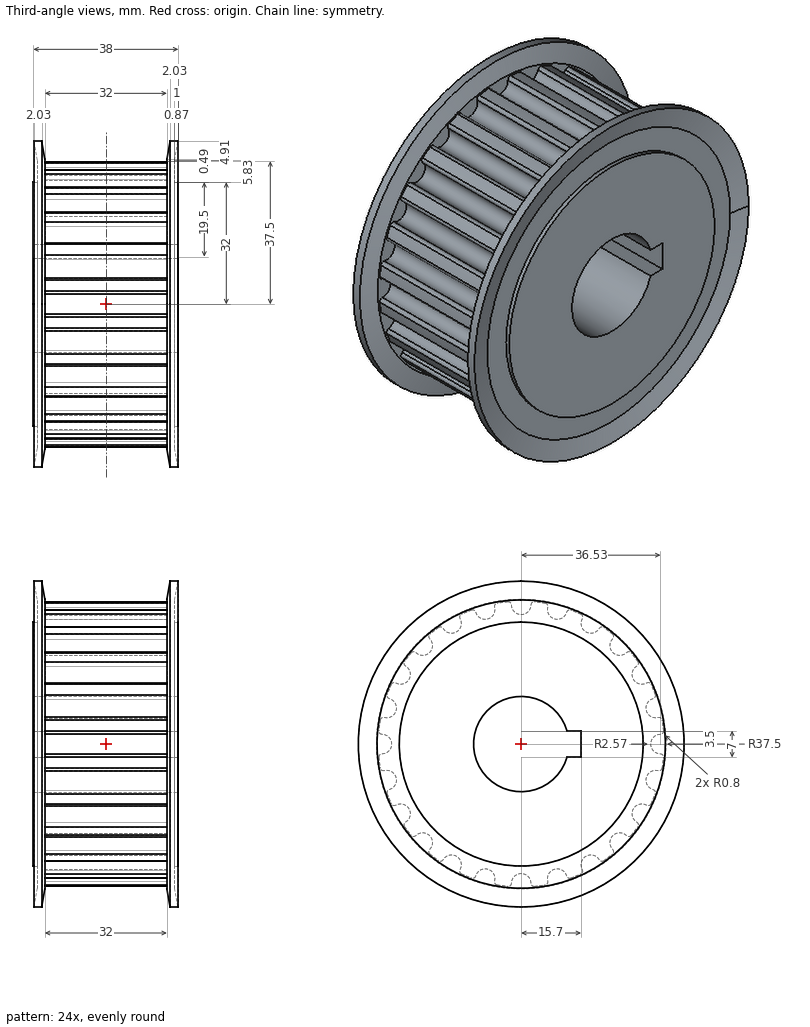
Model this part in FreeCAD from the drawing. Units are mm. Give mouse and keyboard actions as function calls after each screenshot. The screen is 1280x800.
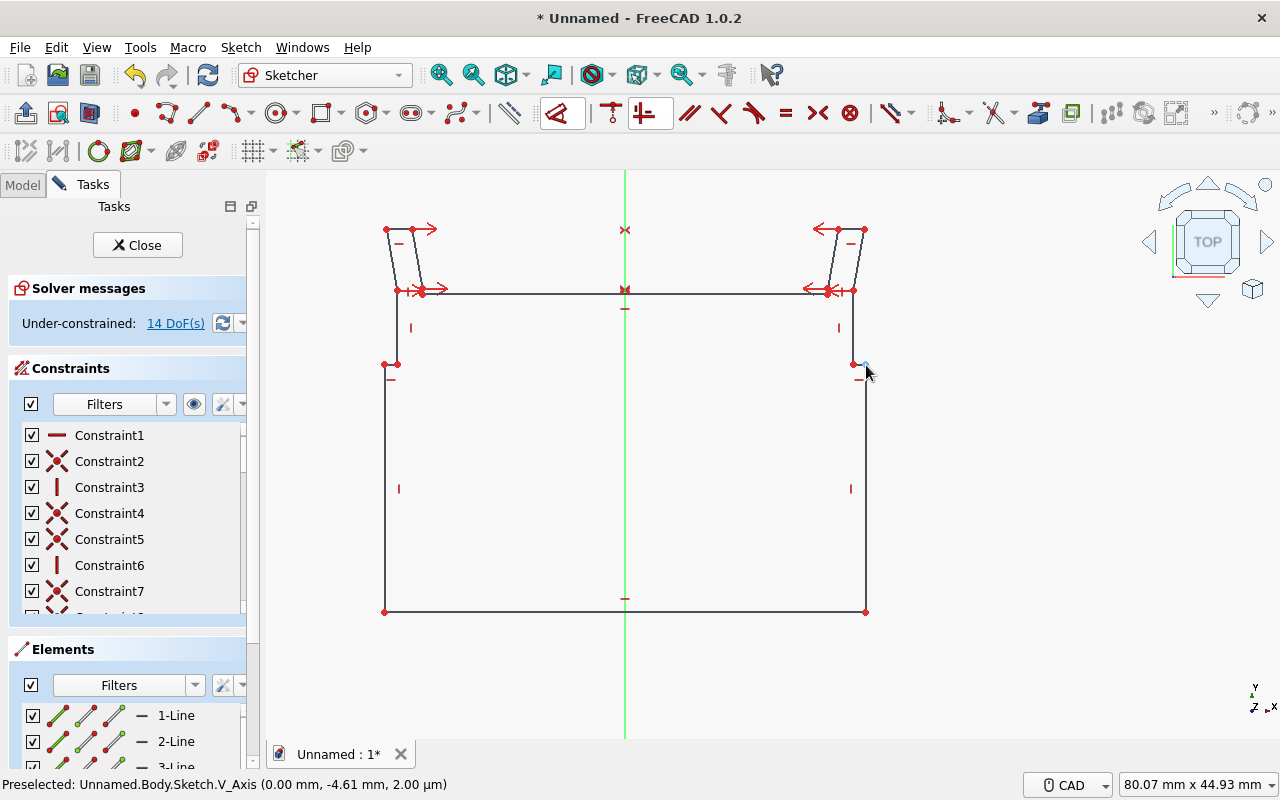
click(866, 365)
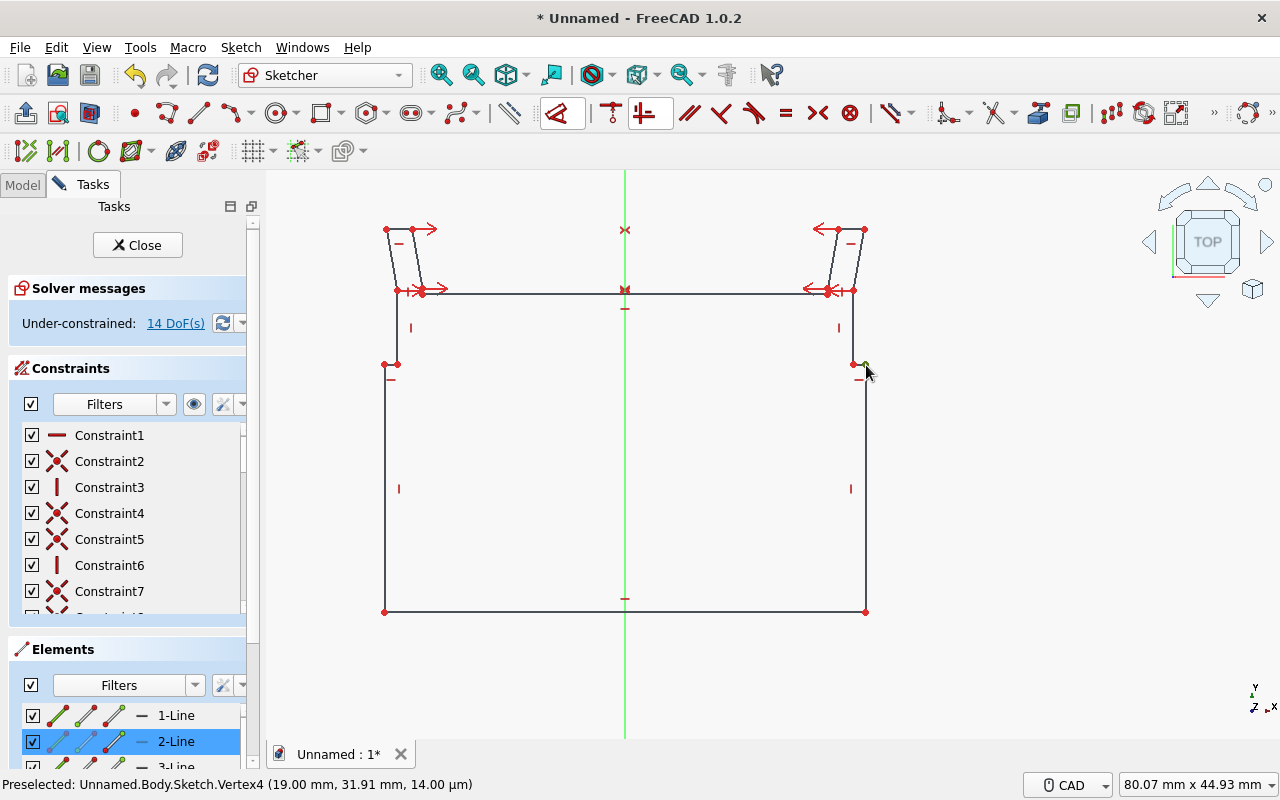
click(385, 365)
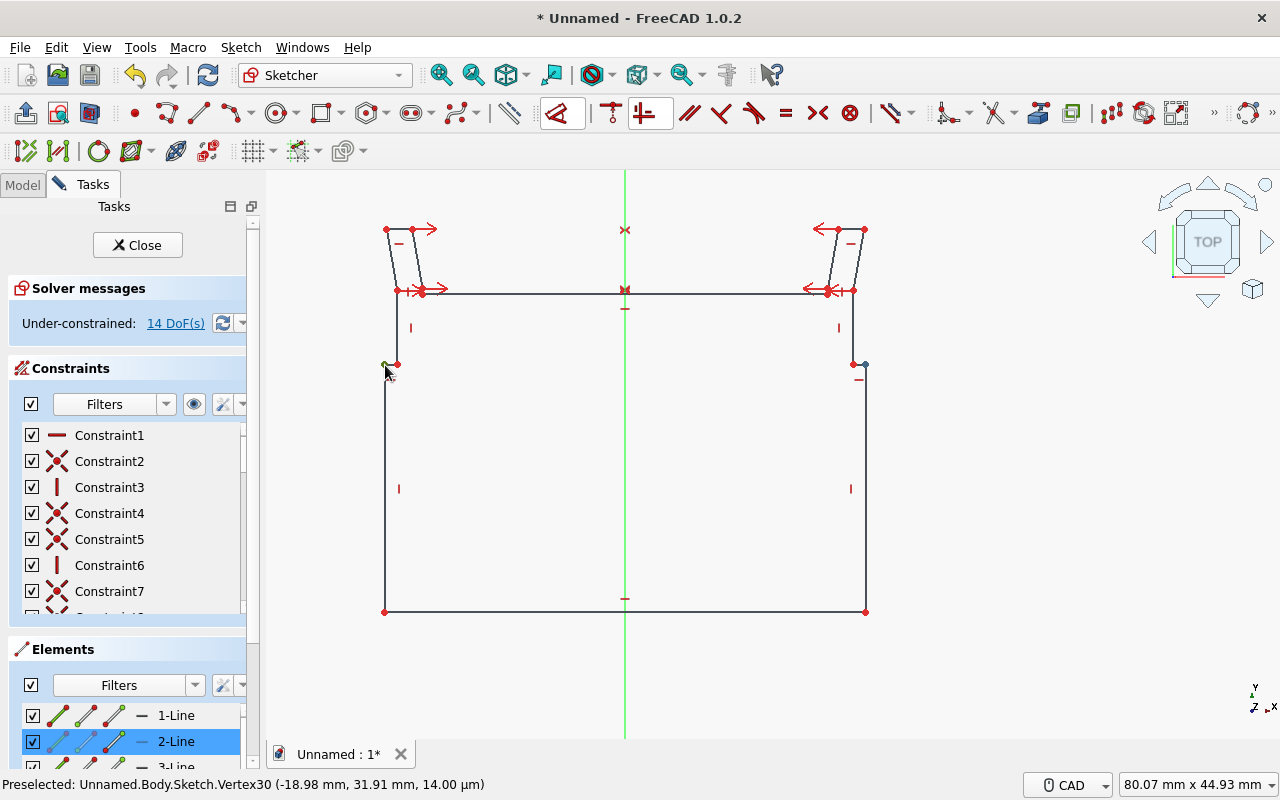
click(625, 674)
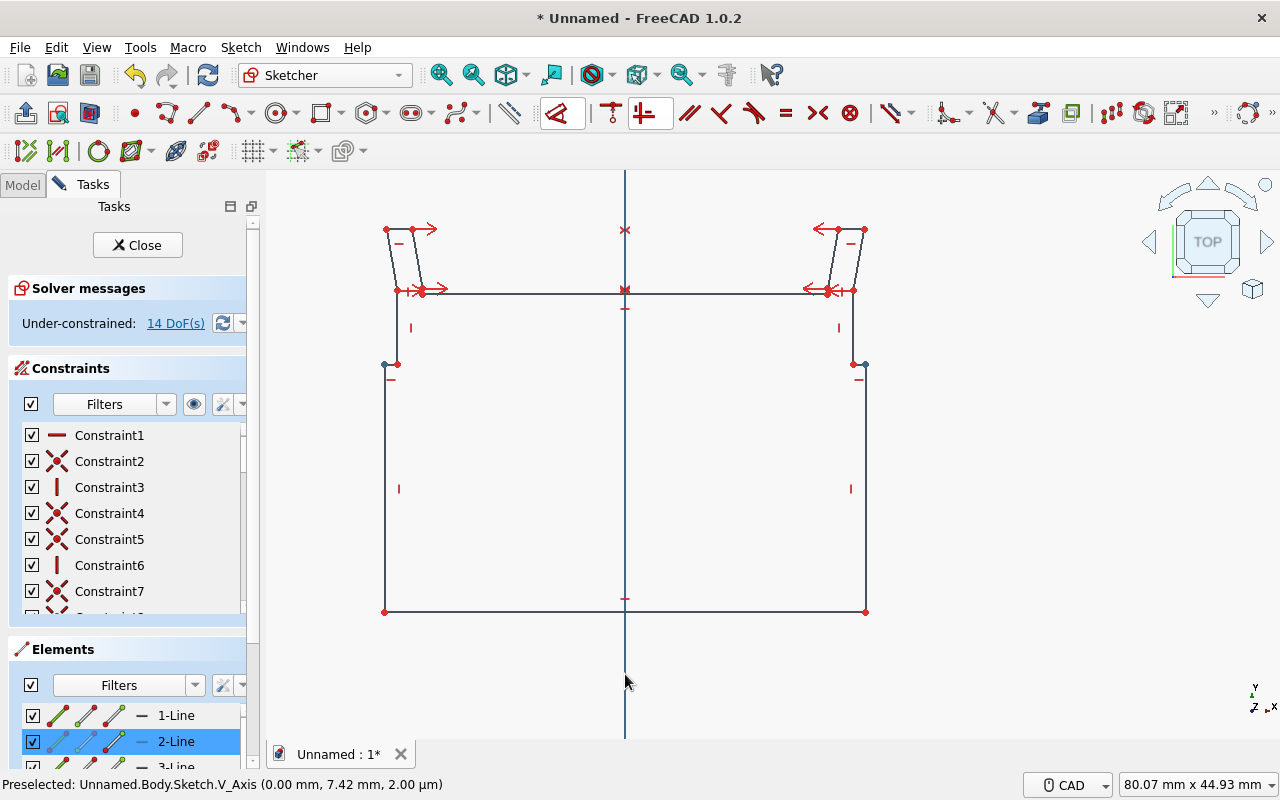
click(818, 114)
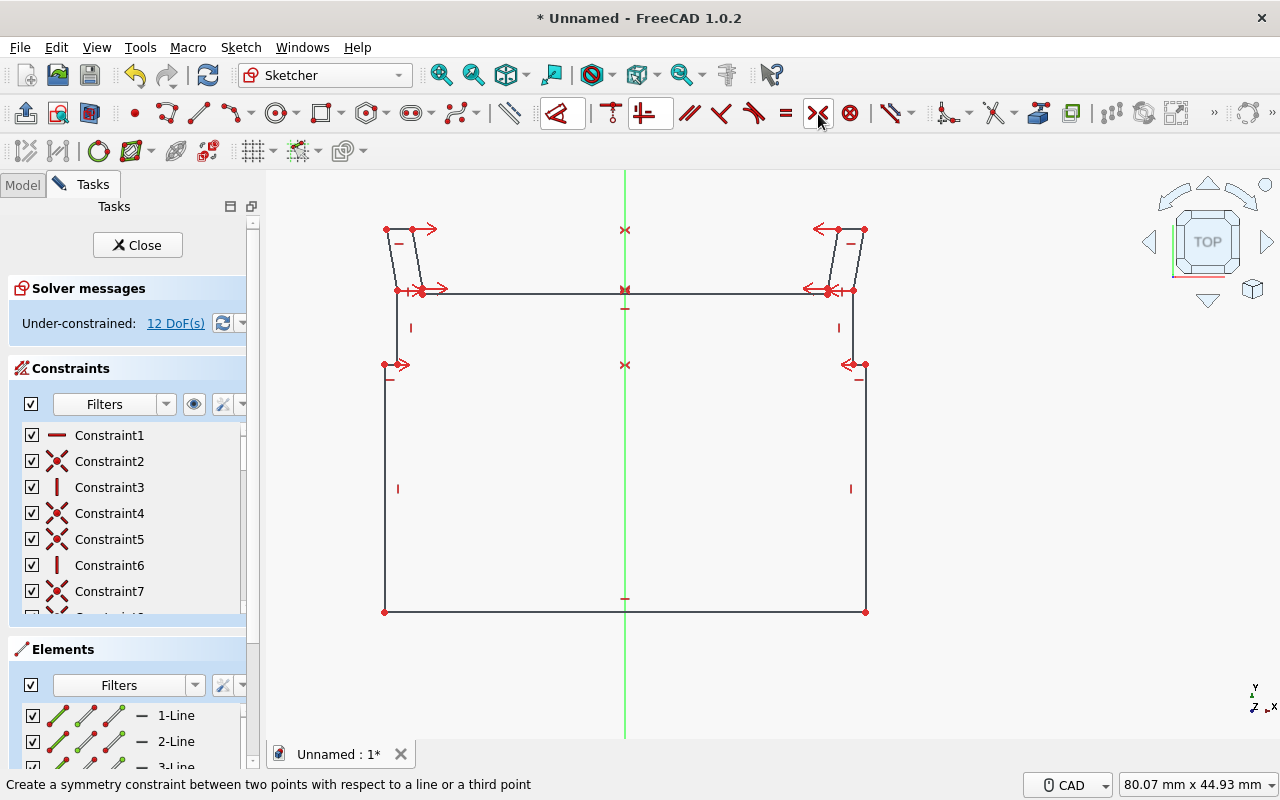
click(556, 114)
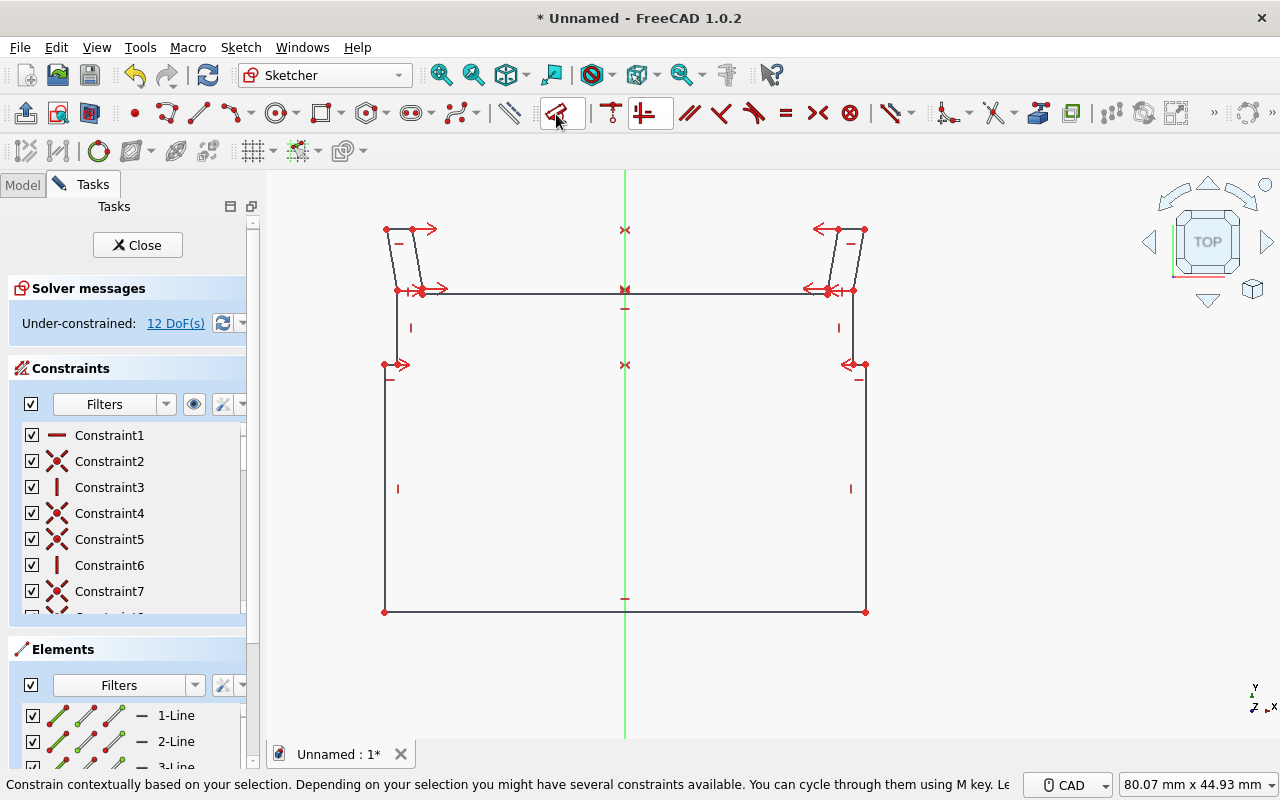
scroll(860, 365, up, 6)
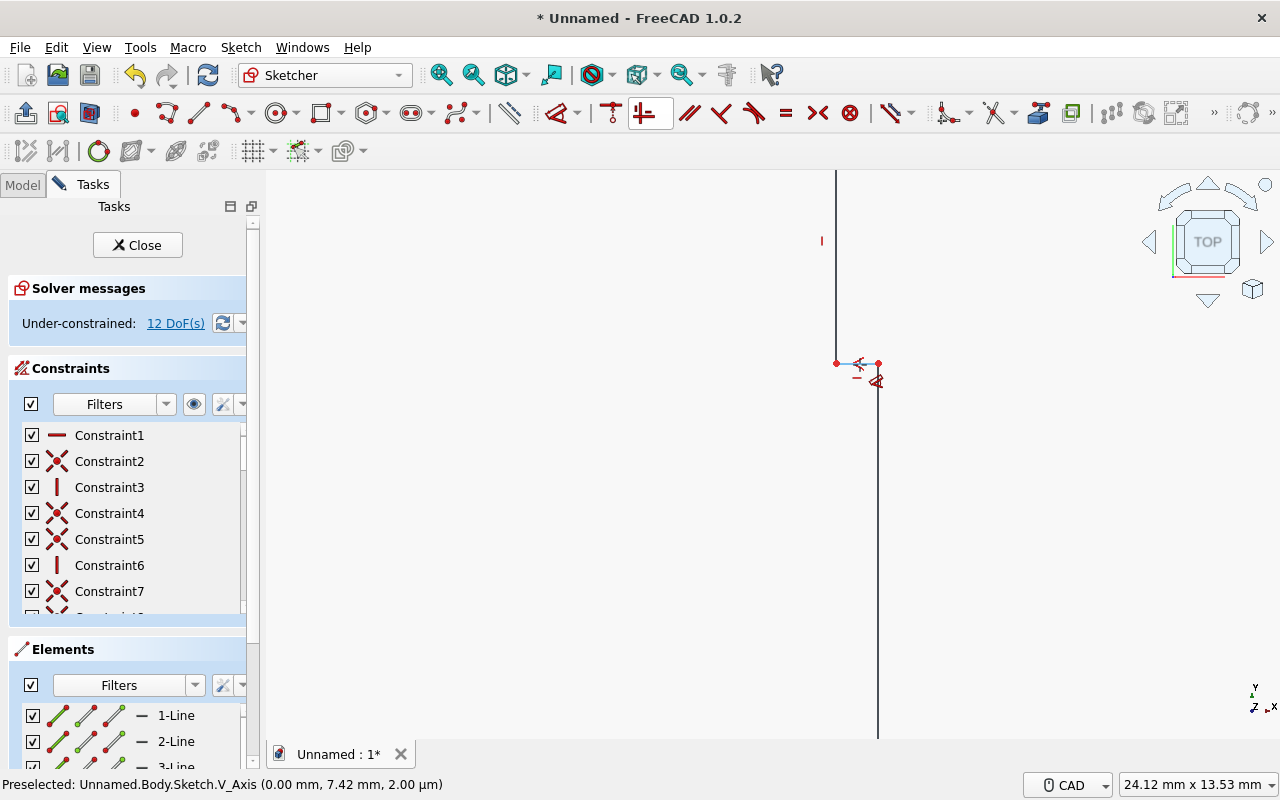
click(857, 364)
click(857, 330)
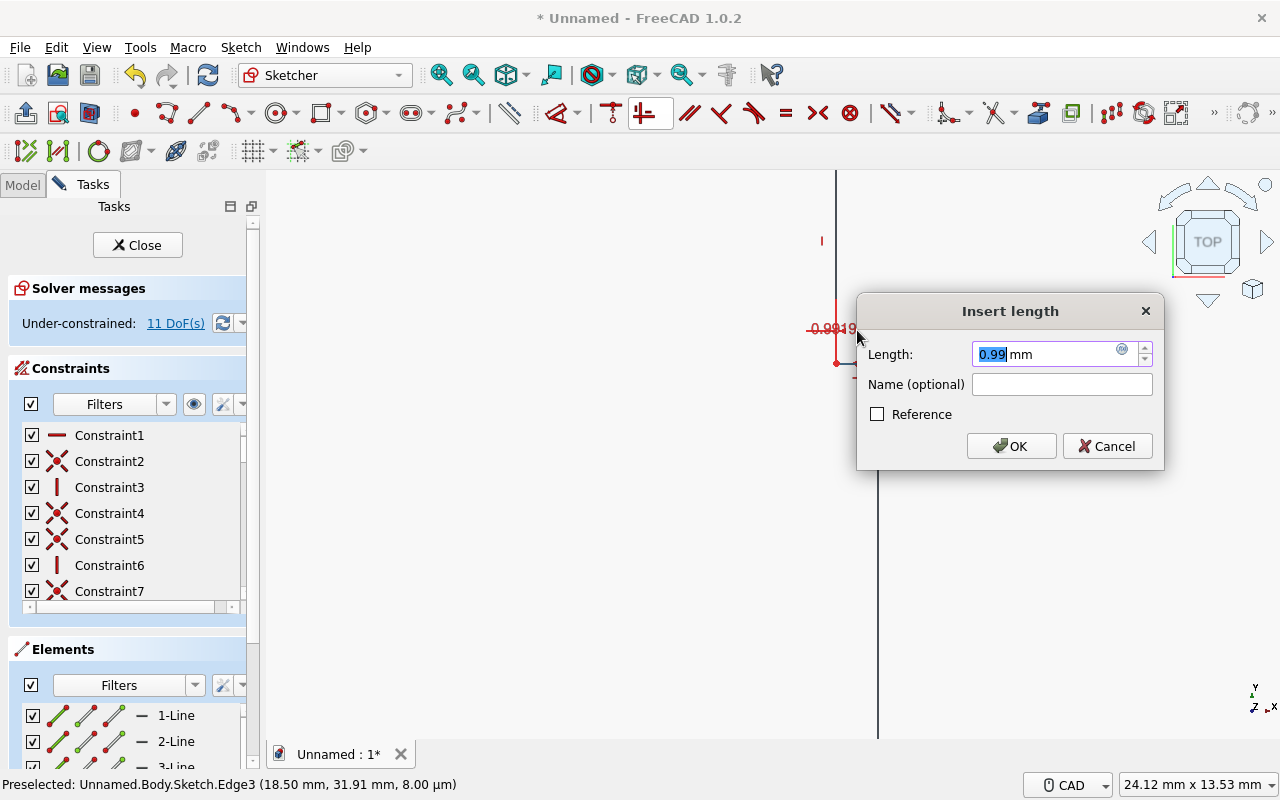
text(1)
key(Return)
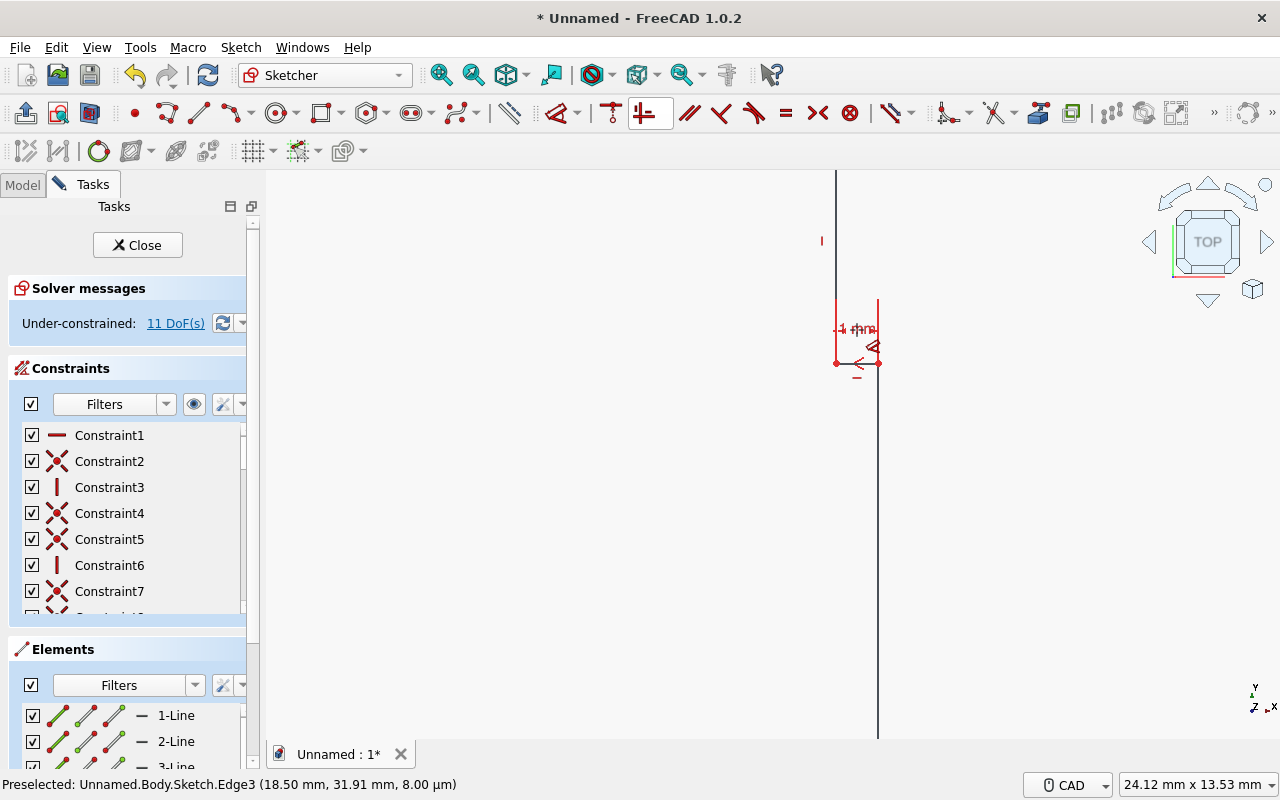
scroll(863, 365, down, 8)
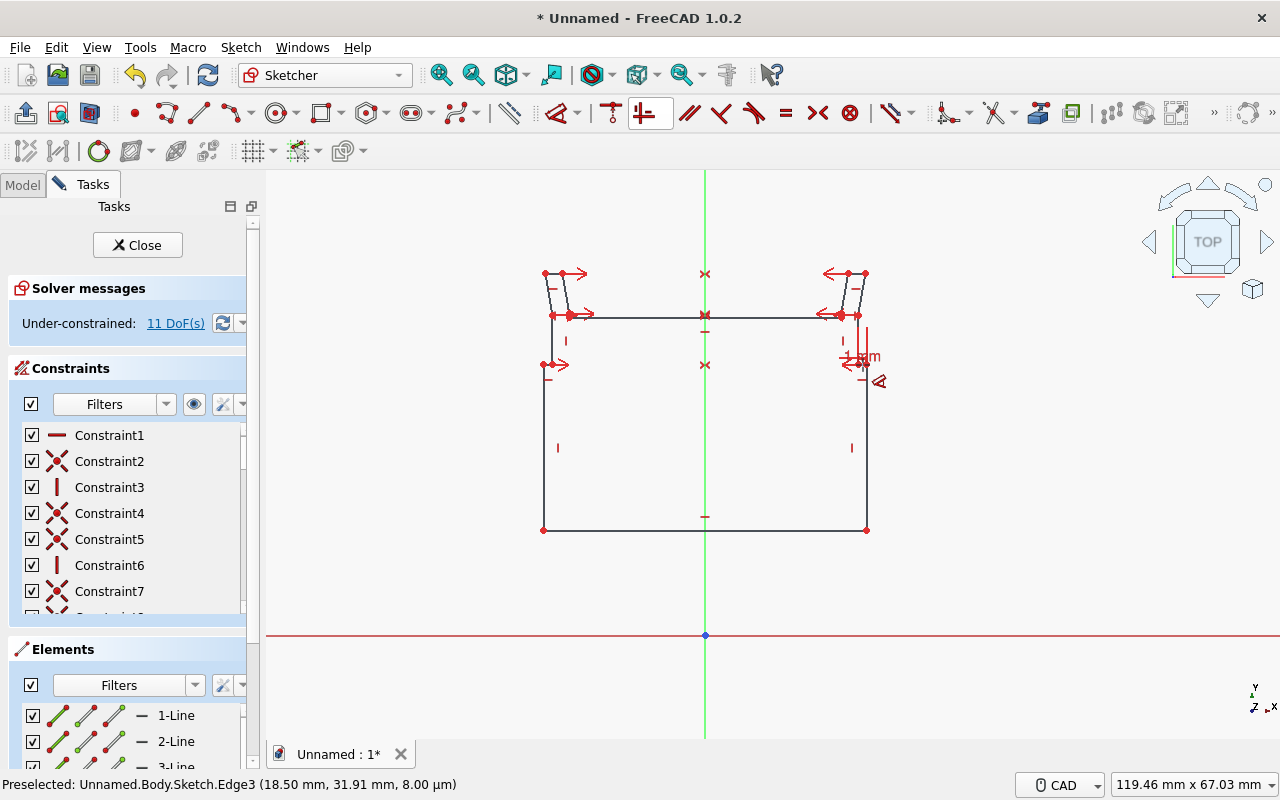
click(641, 531)
click(631, 565)